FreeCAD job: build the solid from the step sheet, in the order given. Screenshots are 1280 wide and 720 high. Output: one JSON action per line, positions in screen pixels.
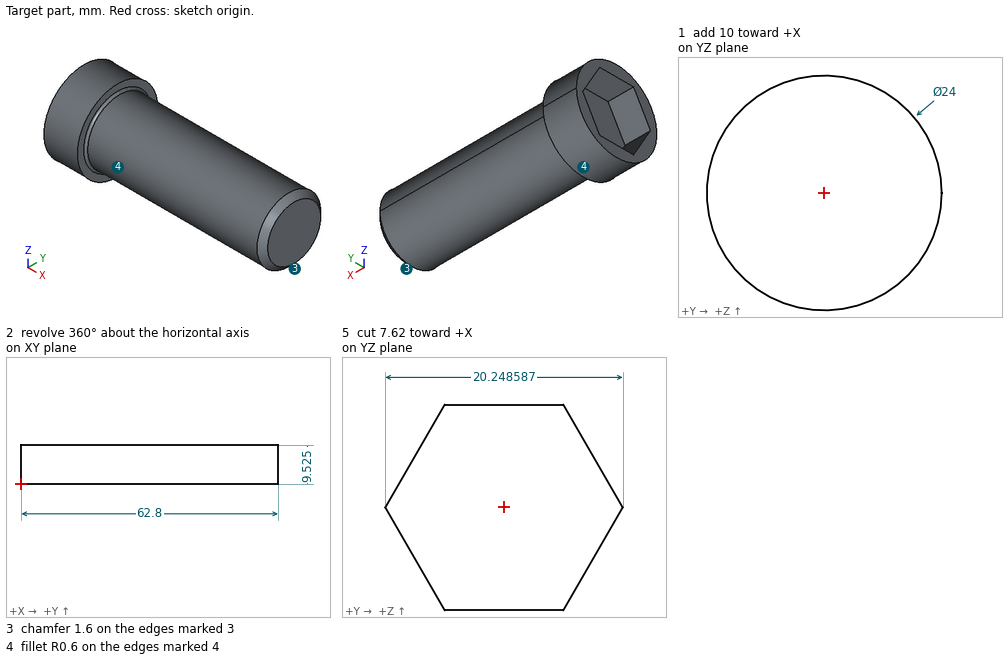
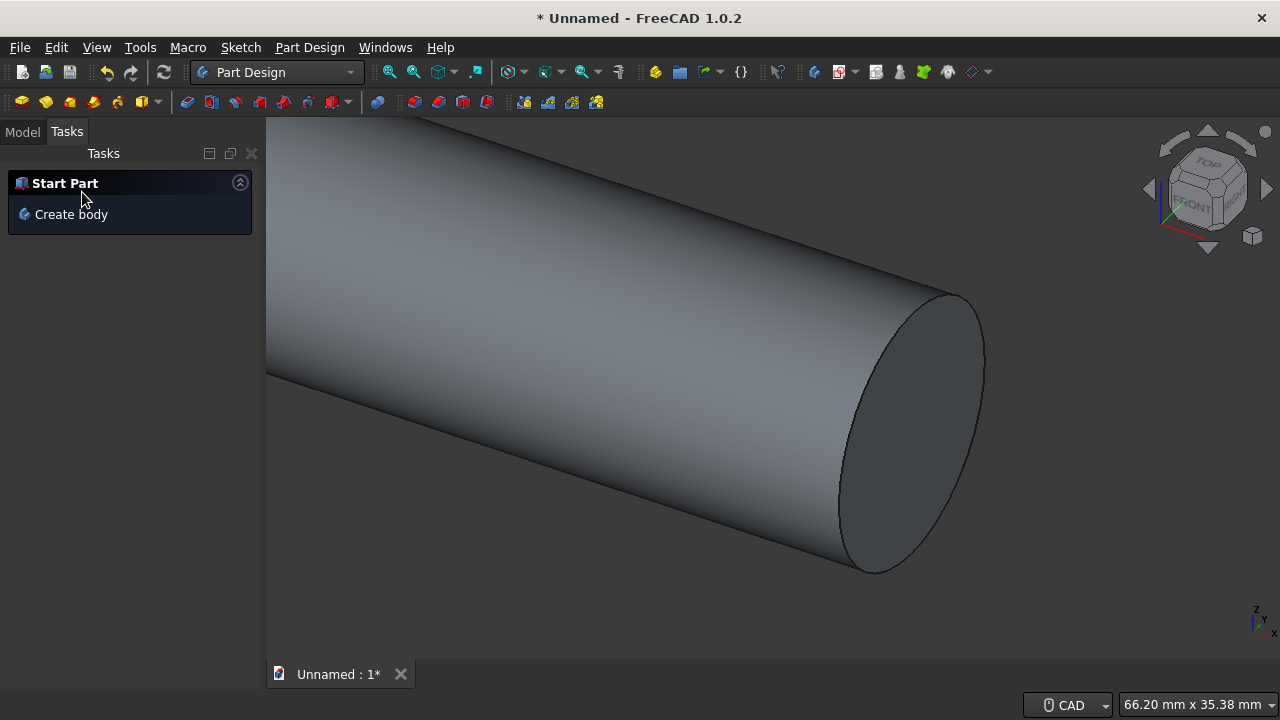
{"action": "left_click", "coordinate": [390, 72]}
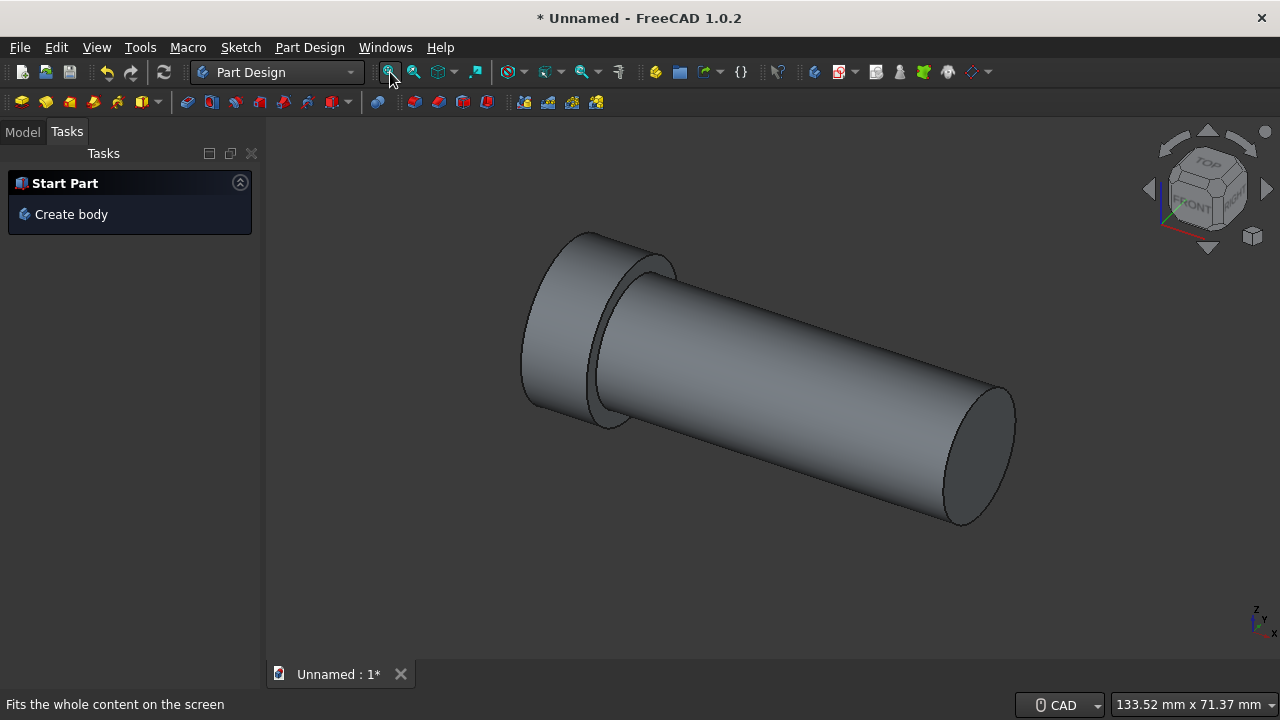
{"action": "left_click", "coordinate": [943, 491]}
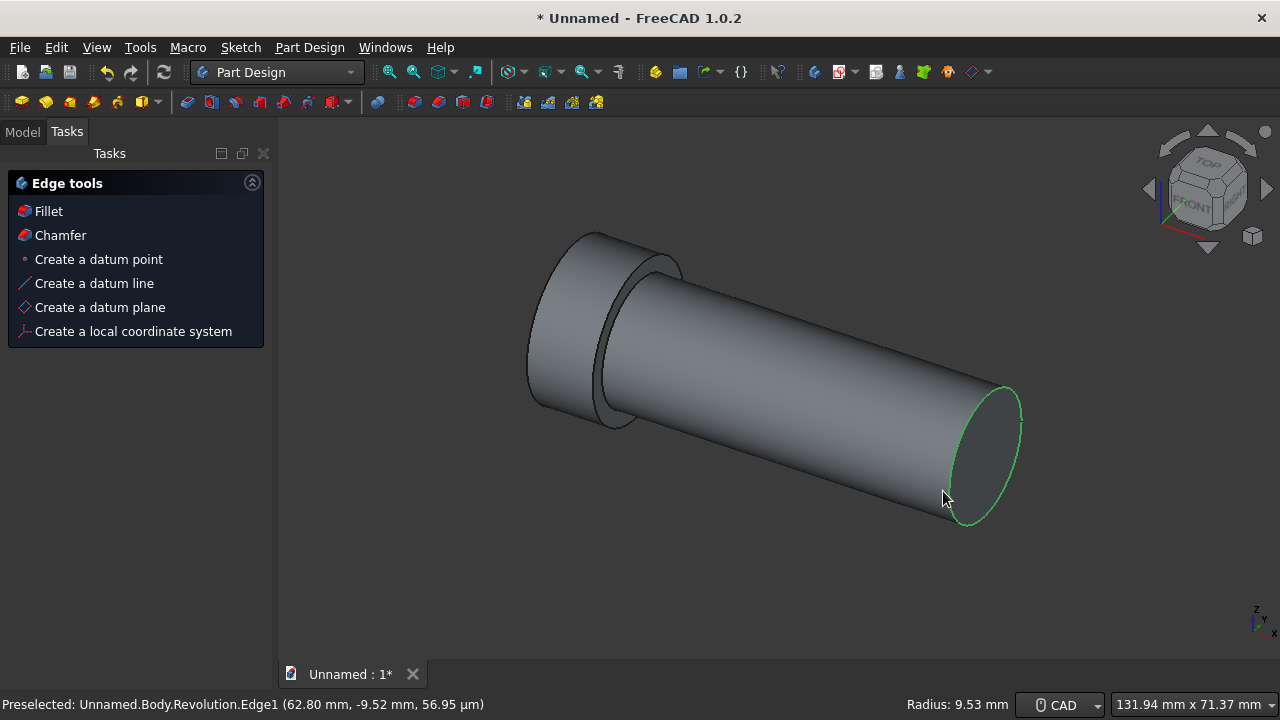
{"action": "left_click", "coordinate": [440, 102]}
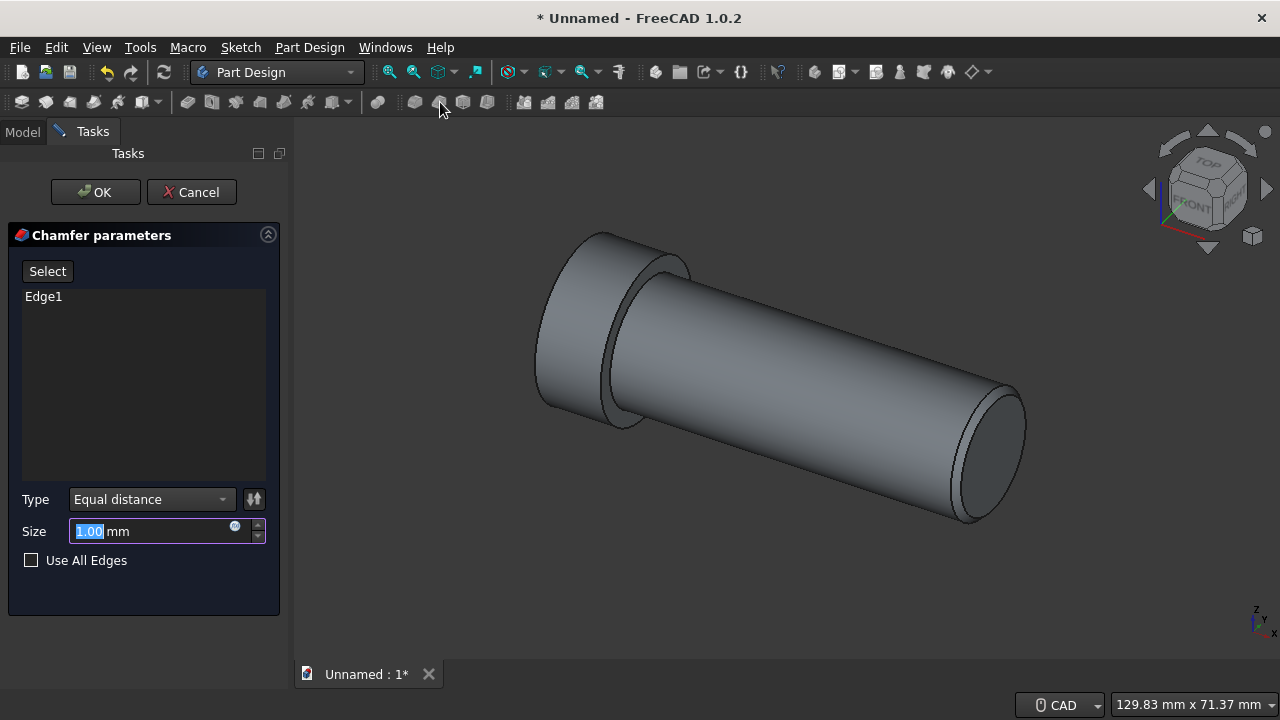
{"action": "type", "text": "1.6"}
{"action": "key", "text": "Tab"}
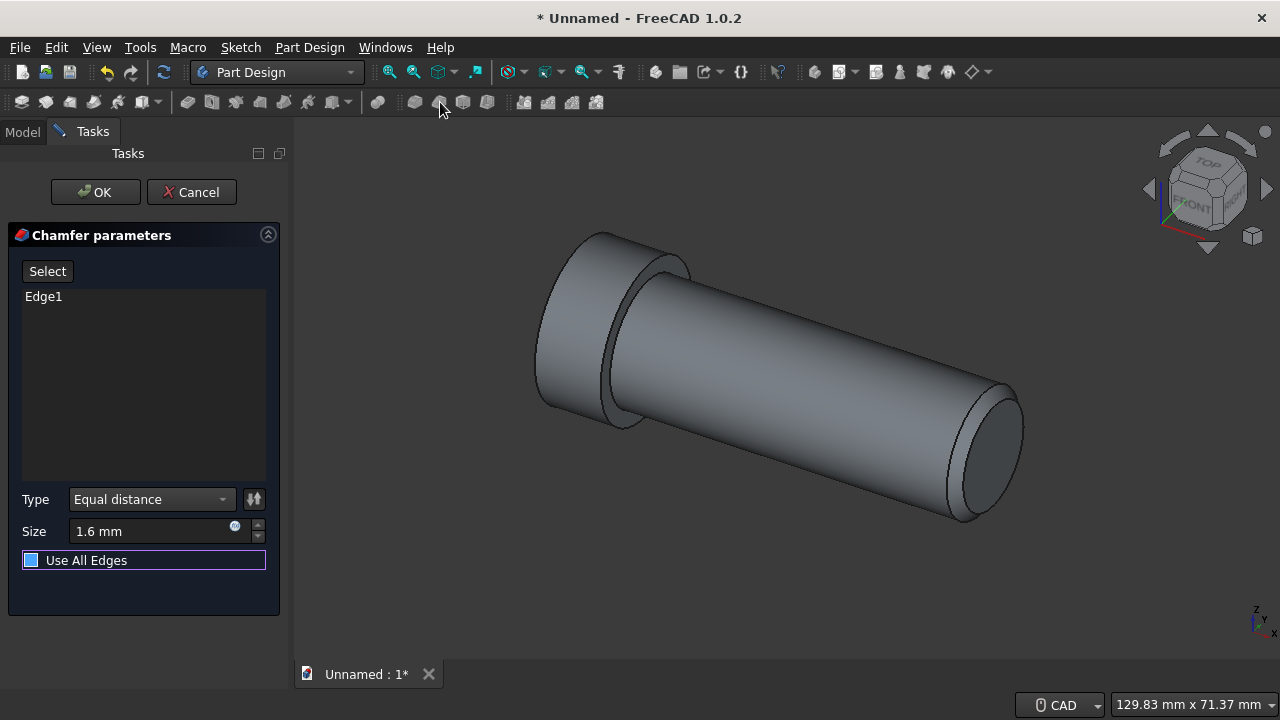
{"action": "left_click", "coordinate": [96, 192]}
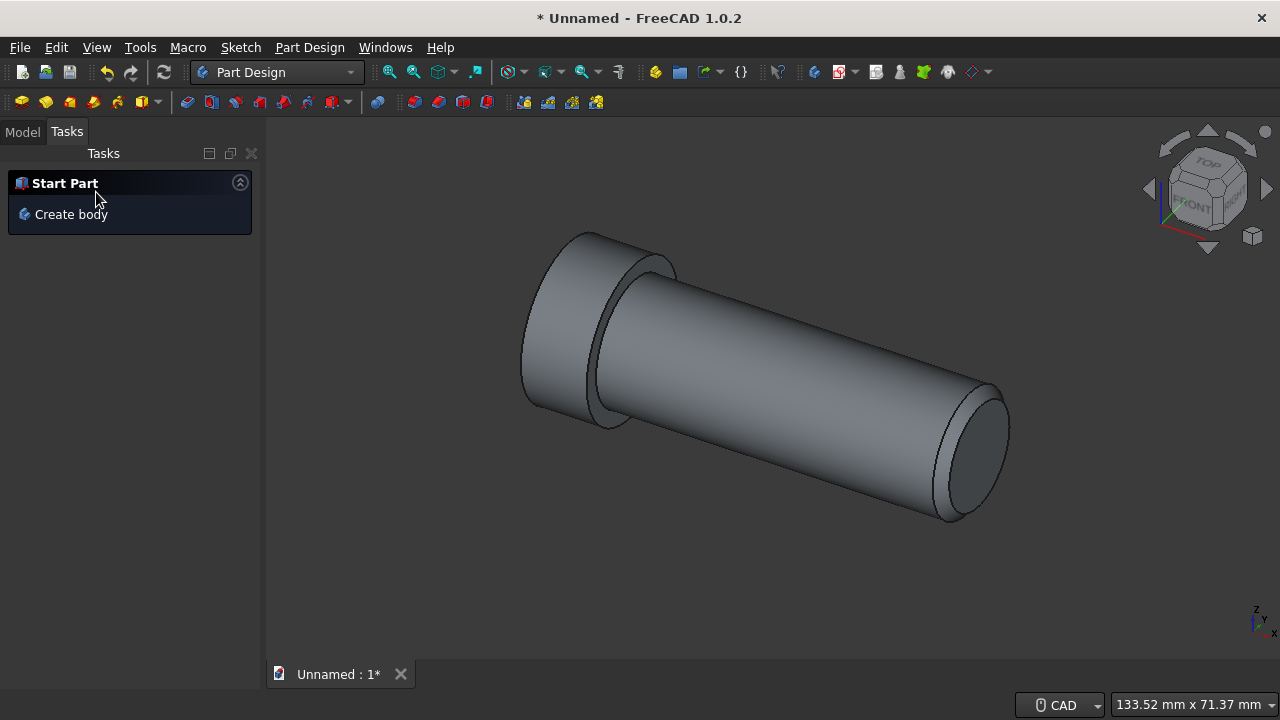
{"action": "key", "text": "0"}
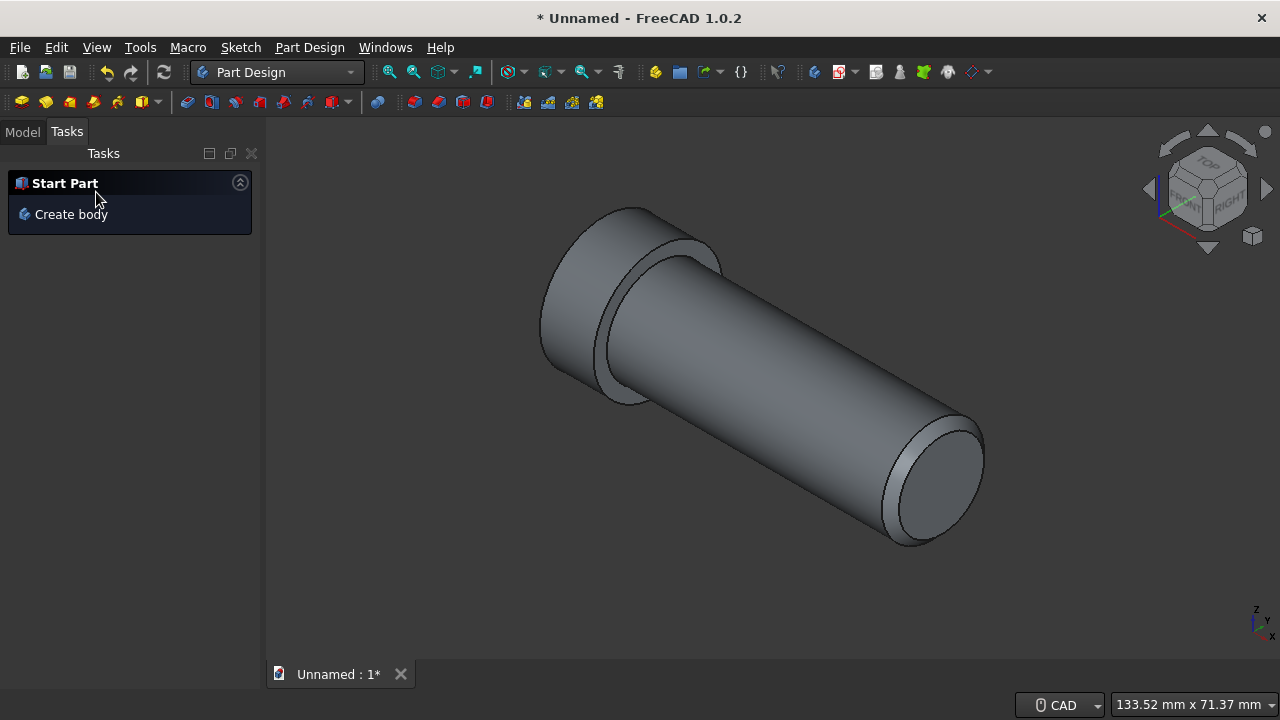
{"action": "key", "text": "2"}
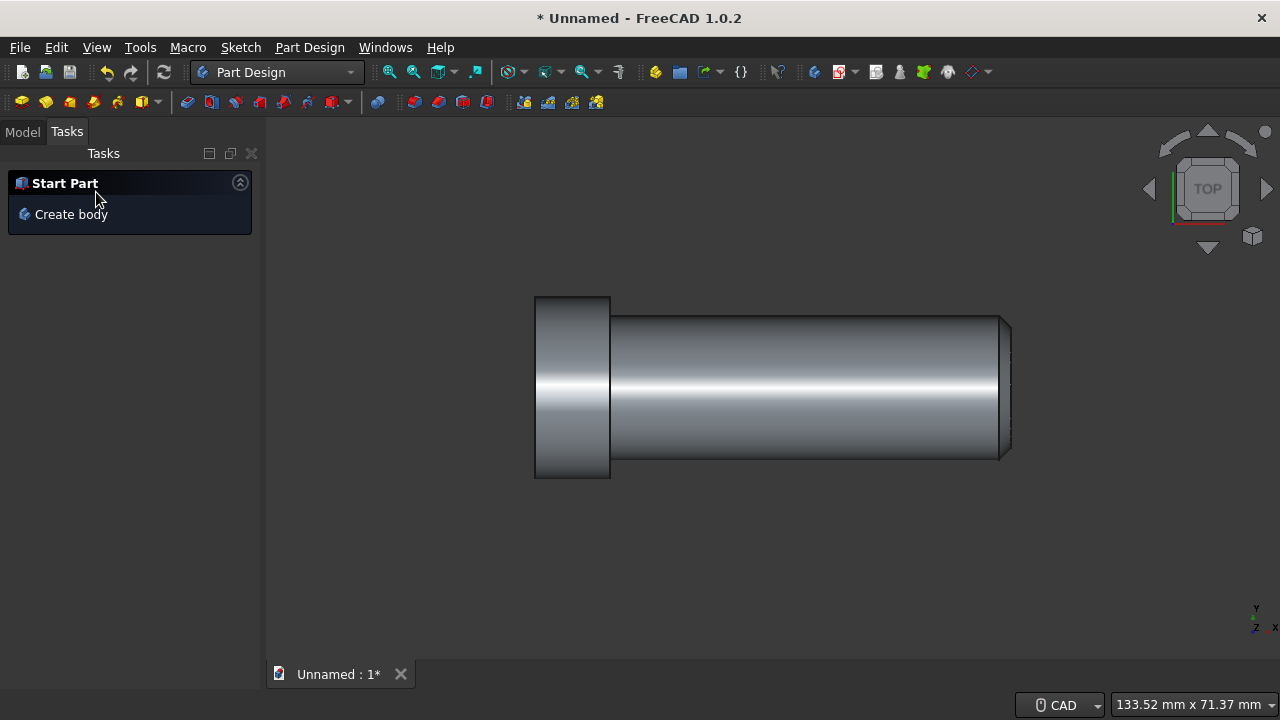
{"action": "key", "text": "1"}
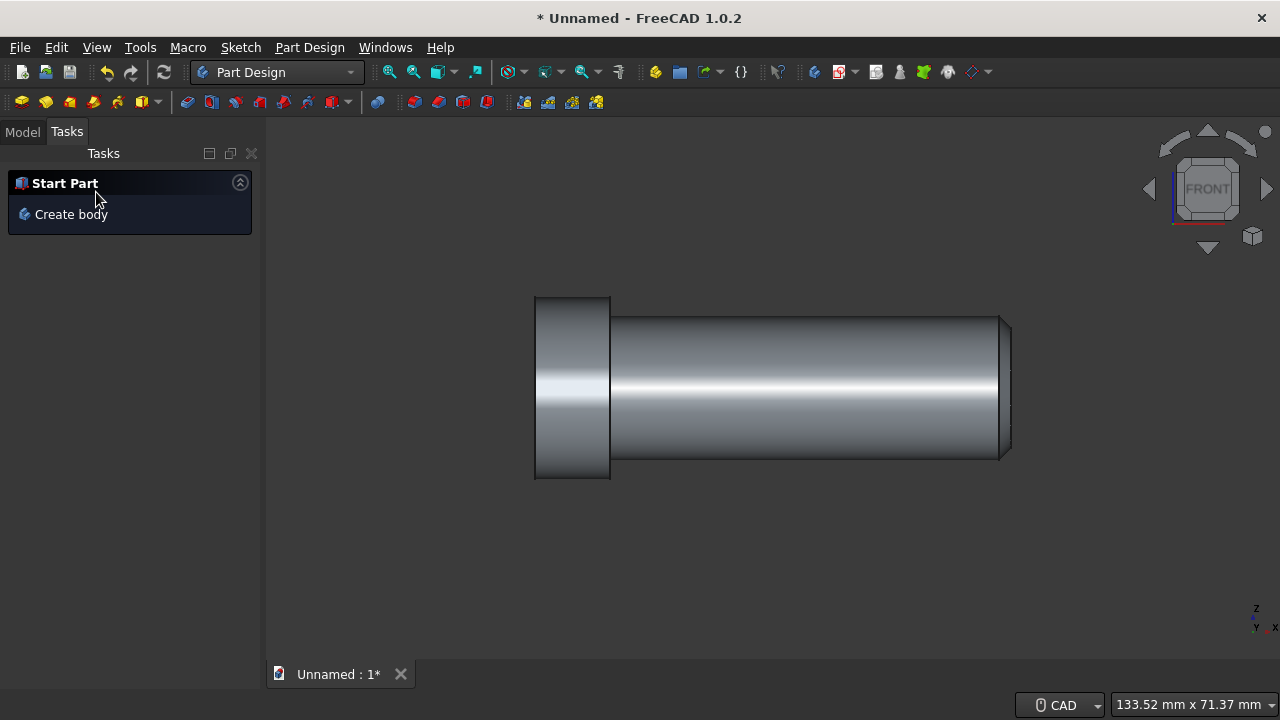
{"action": "key", "text": "3"}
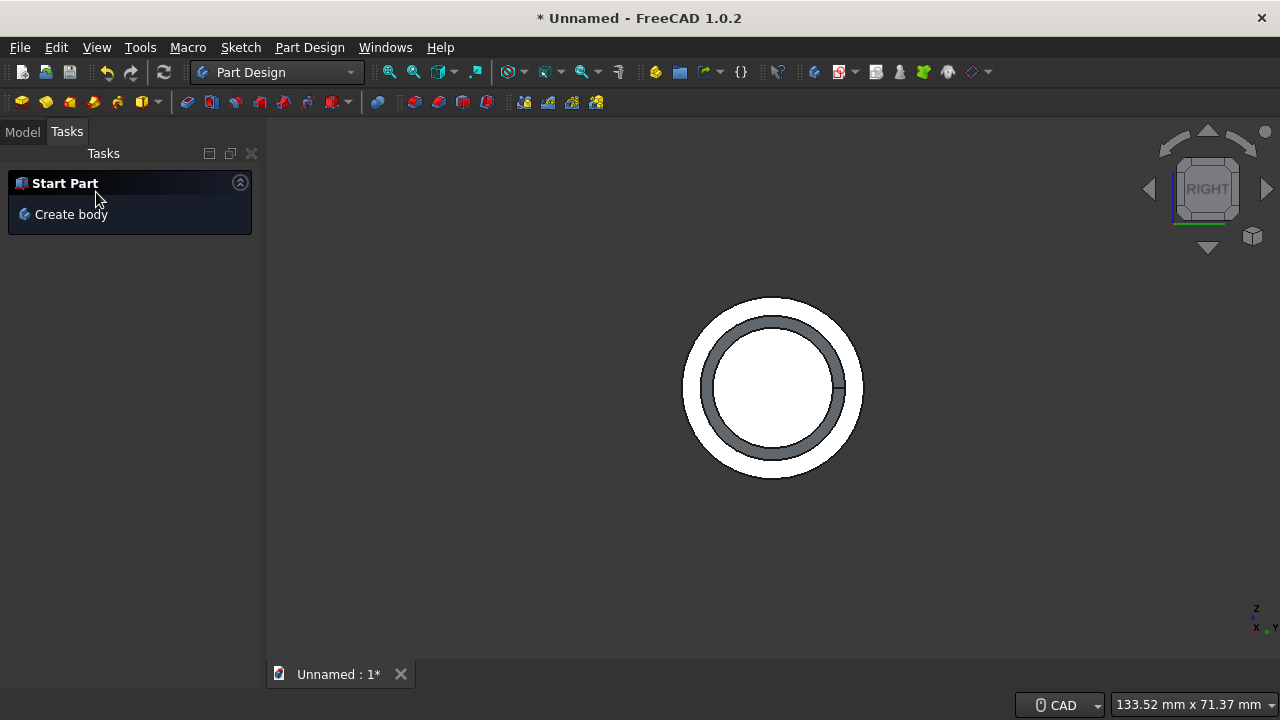
{"action": "left_click", "coordinate": [390, 72]}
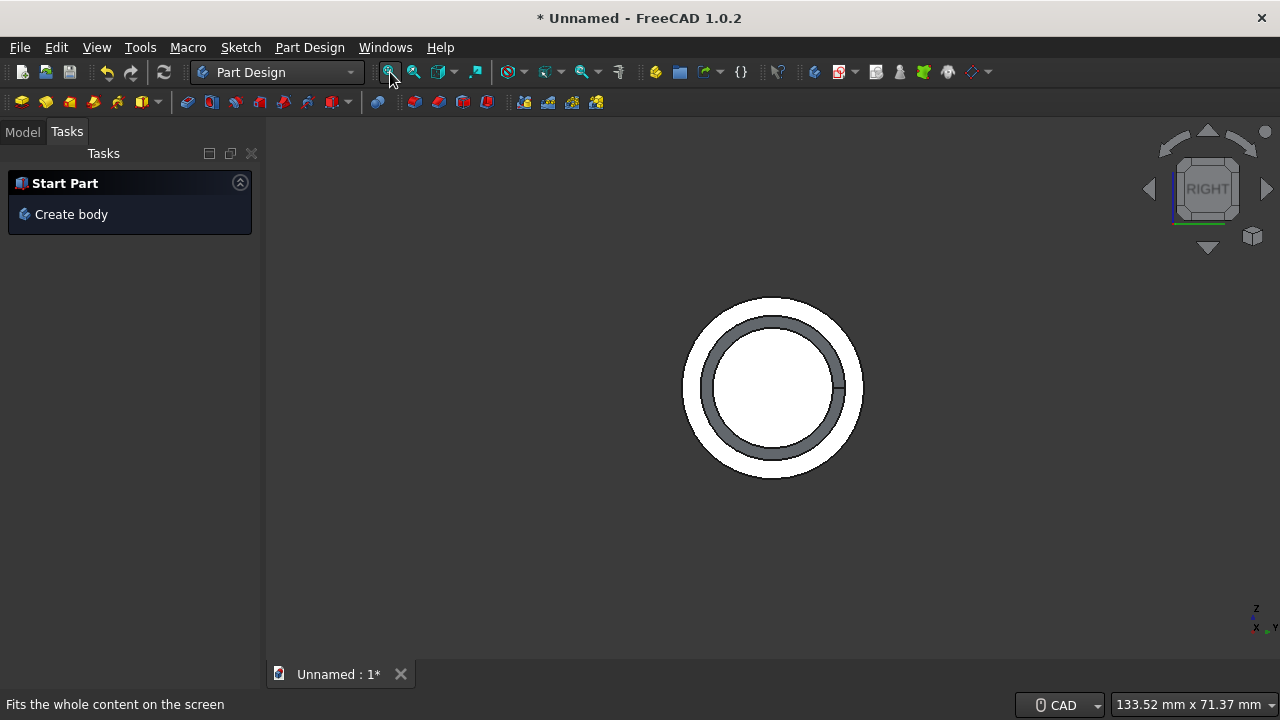
{"action": "key", "text": "5"}